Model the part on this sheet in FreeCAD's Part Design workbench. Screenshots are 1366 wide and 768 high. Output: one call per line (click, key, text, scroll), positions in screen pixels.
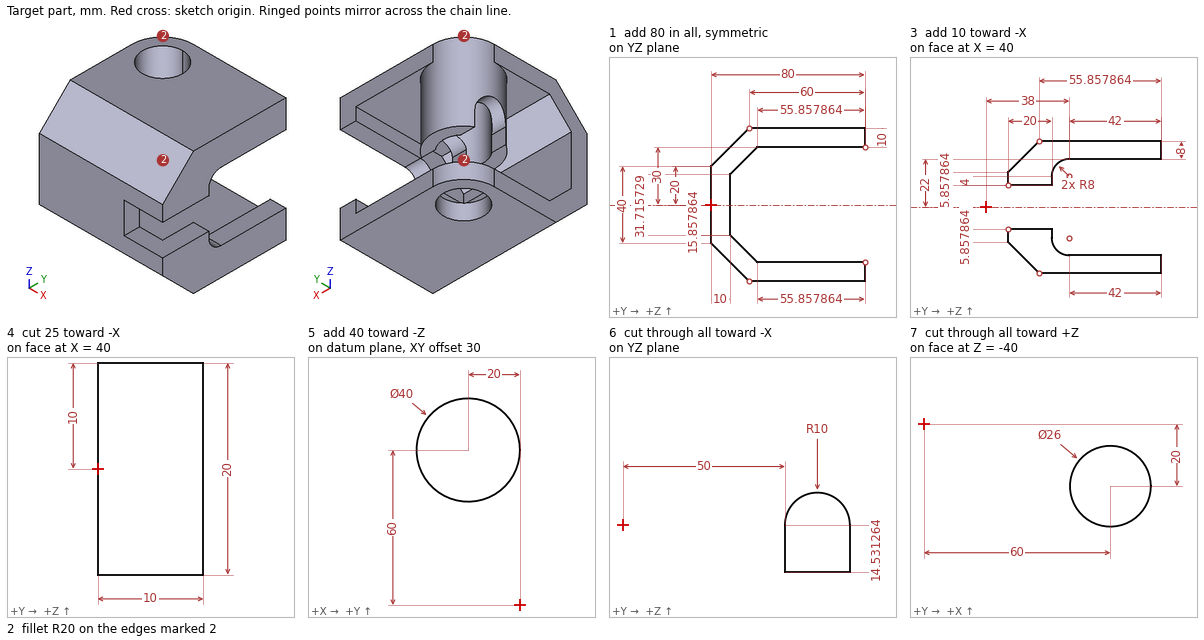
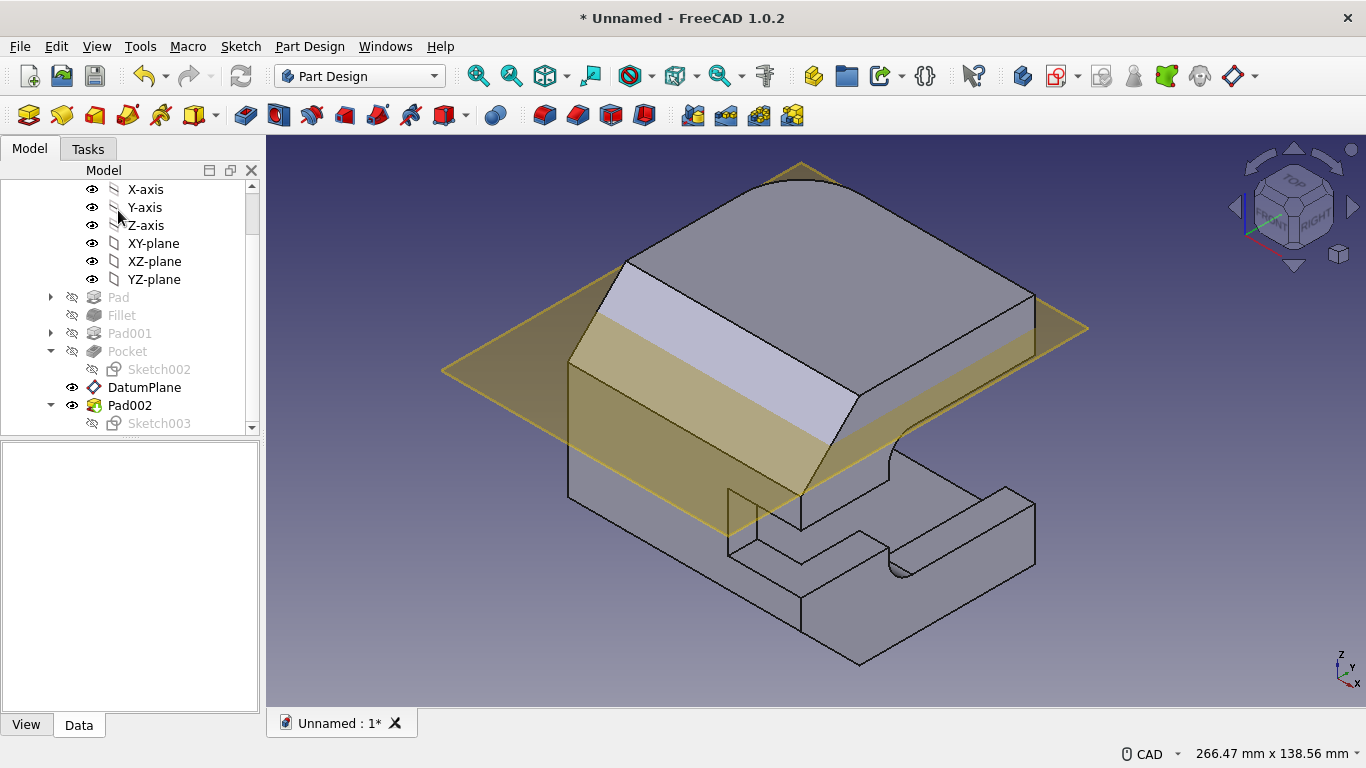
click(117, 387)
key(space)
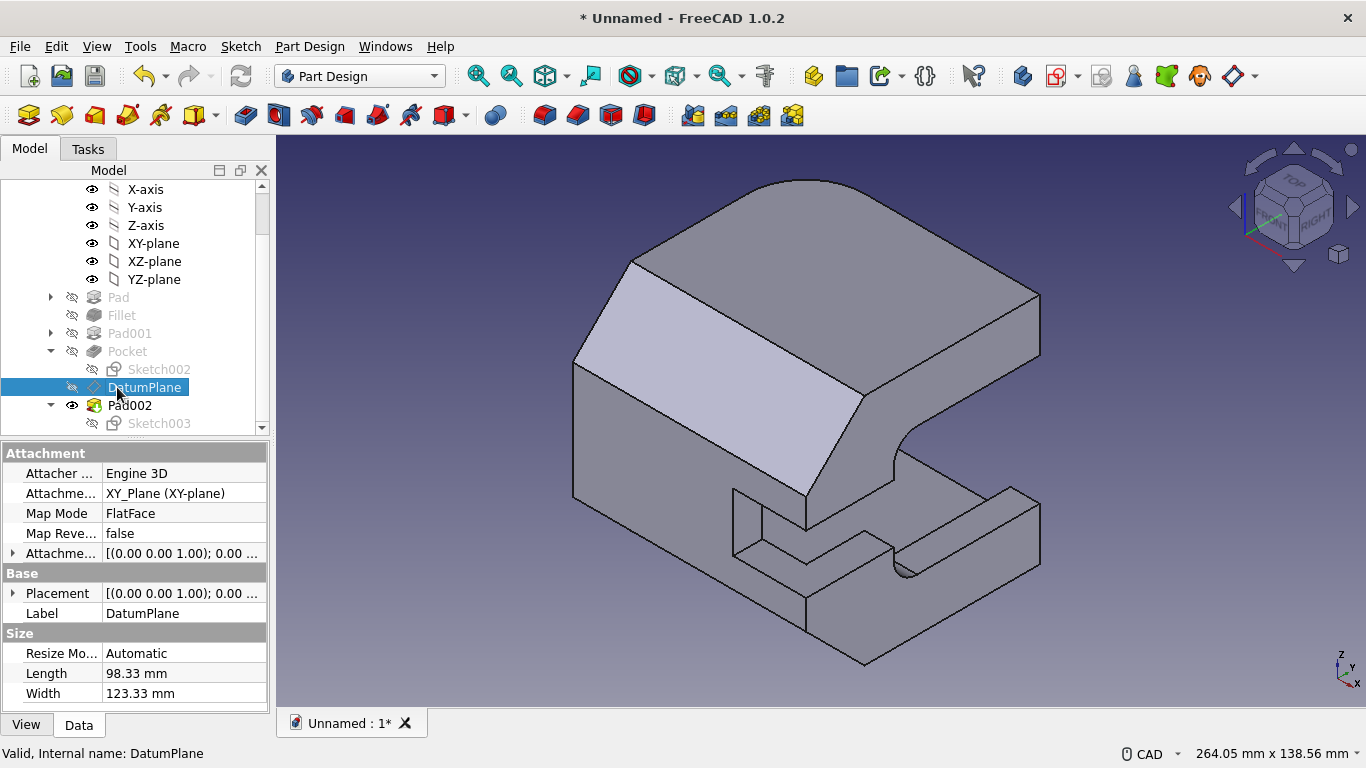
click(316, 667)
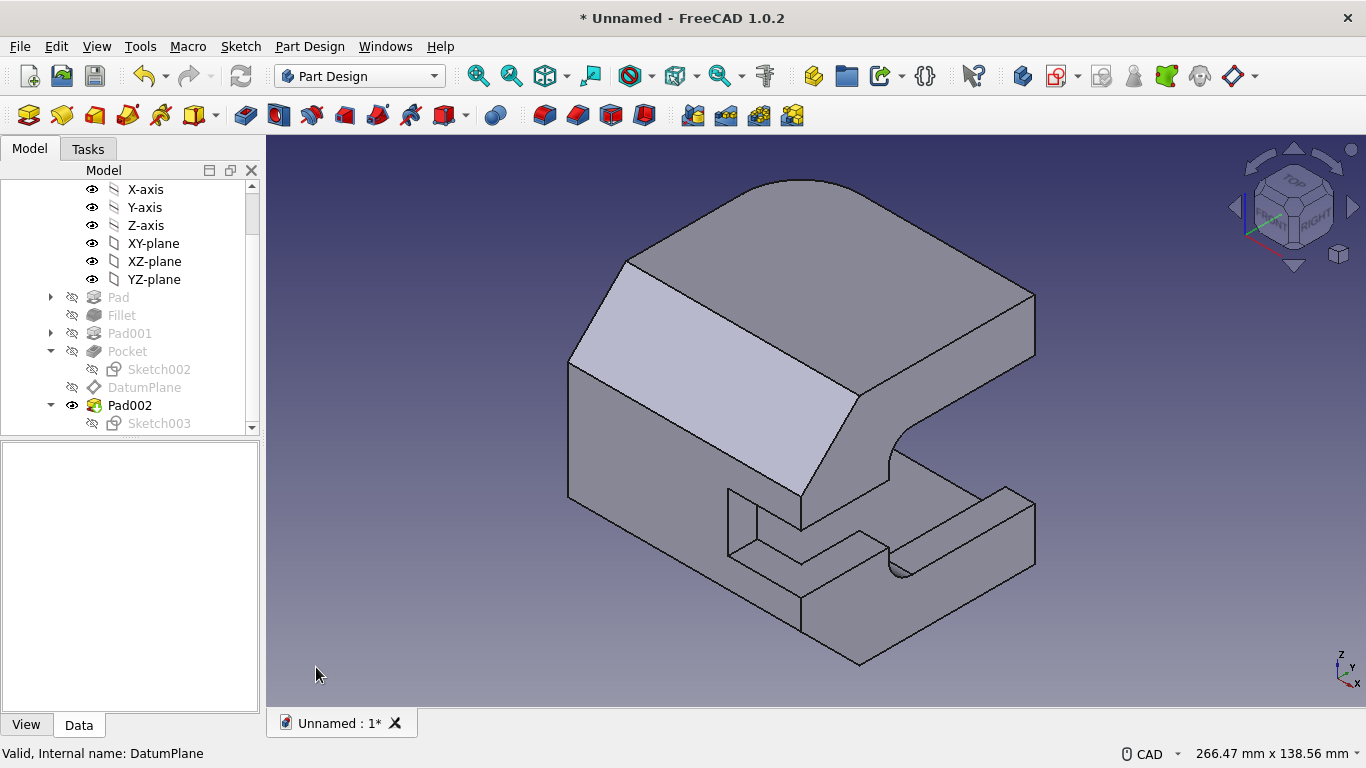
click(1056, 76)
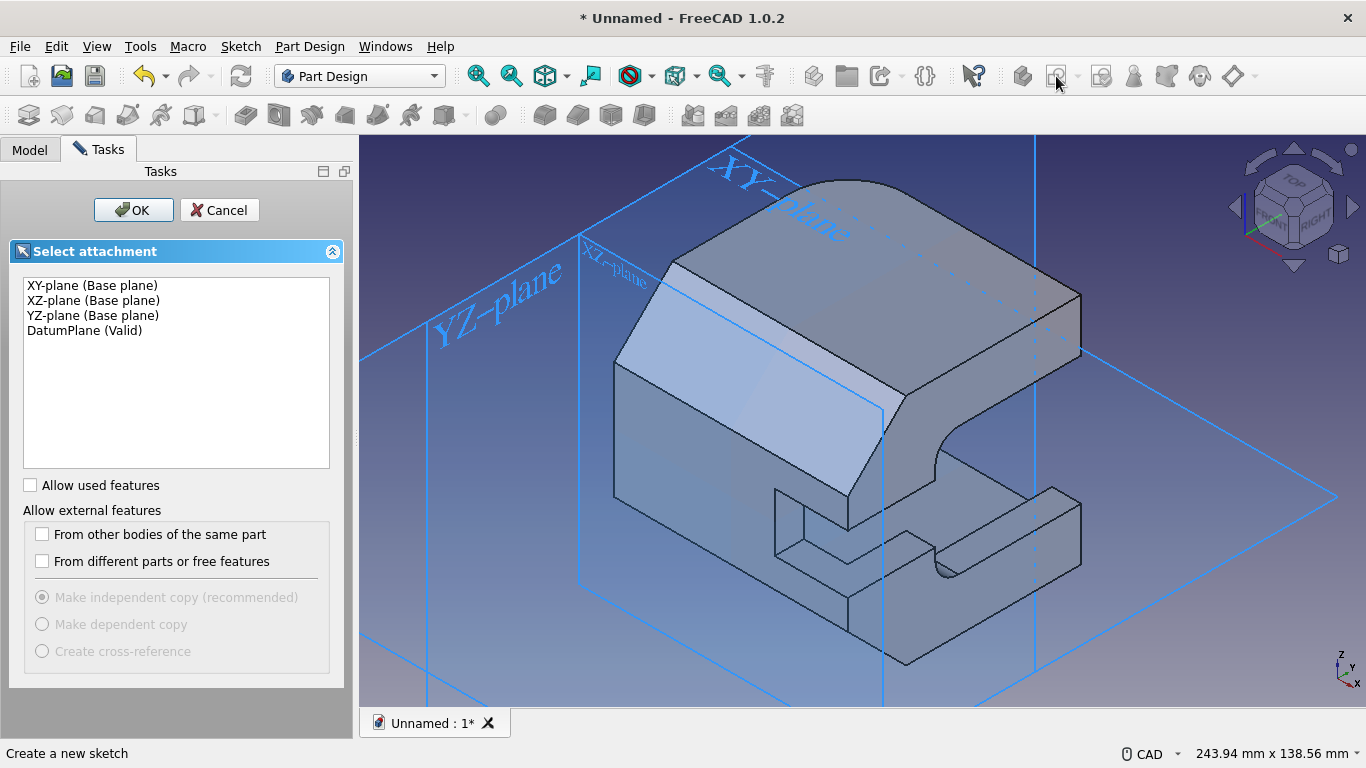
click(84, 316)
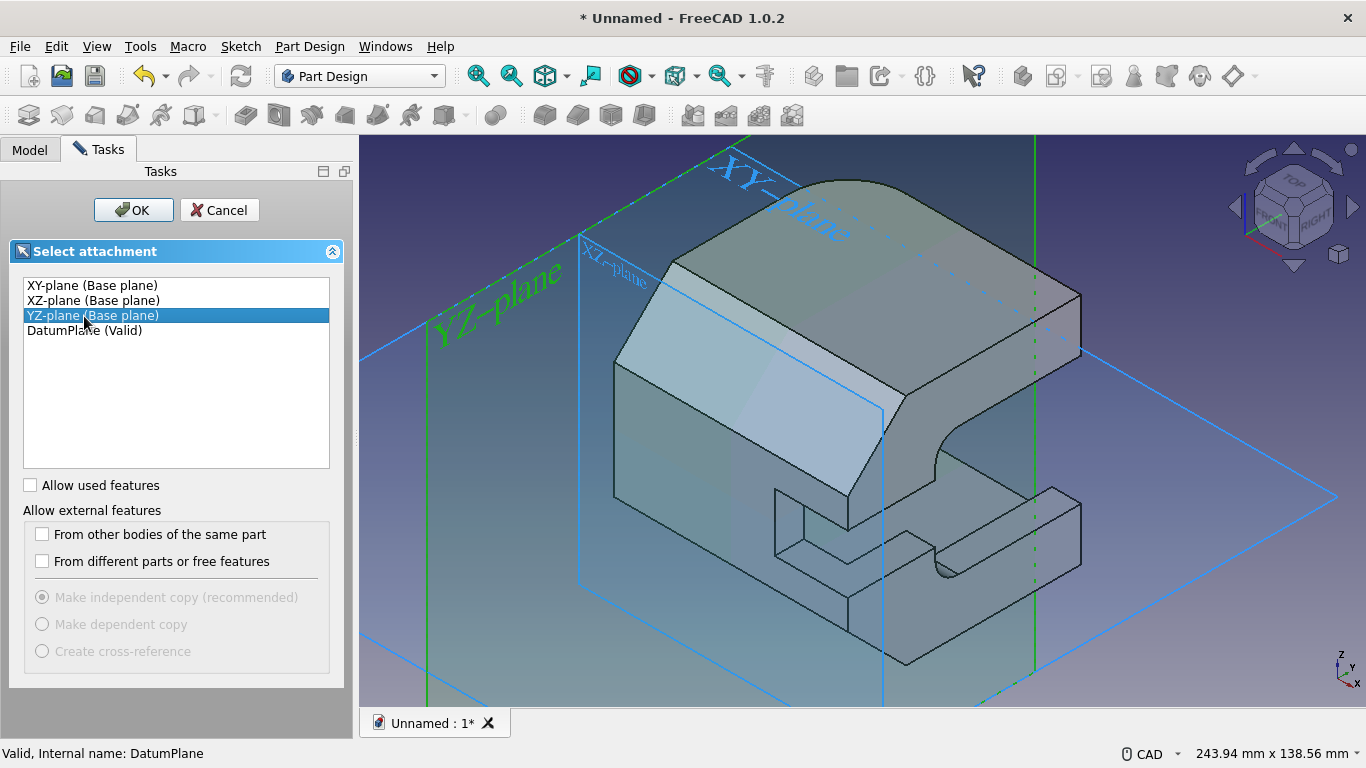
click(134, 210)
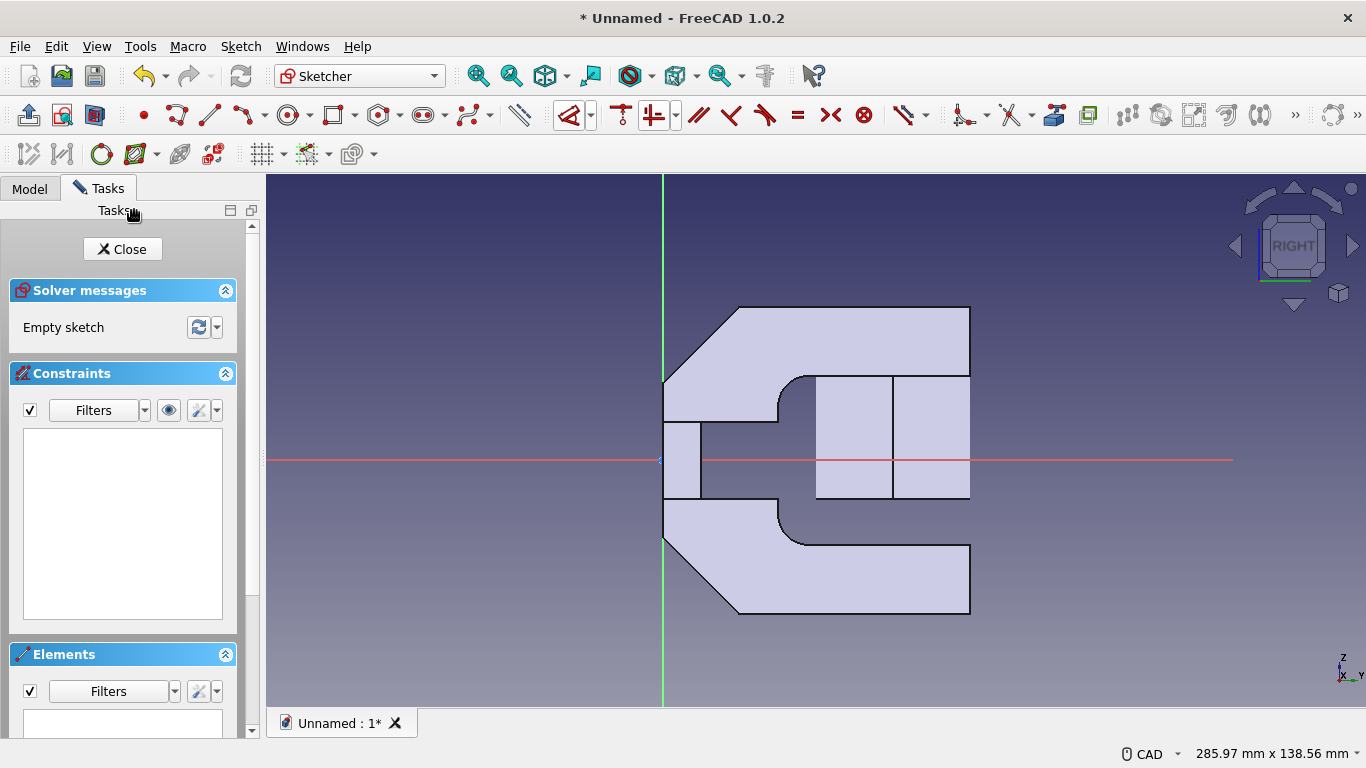
click(95, 116)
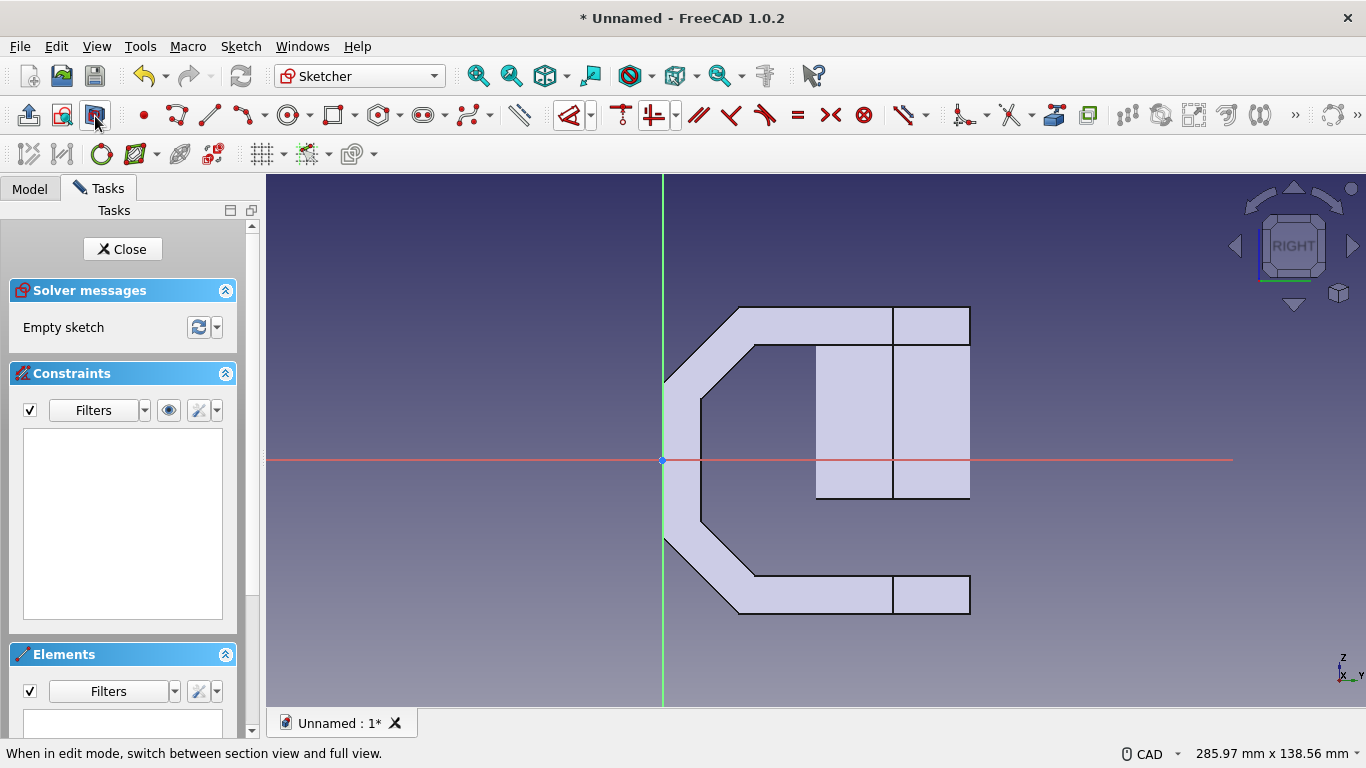
scroll(956, 481, up, 6)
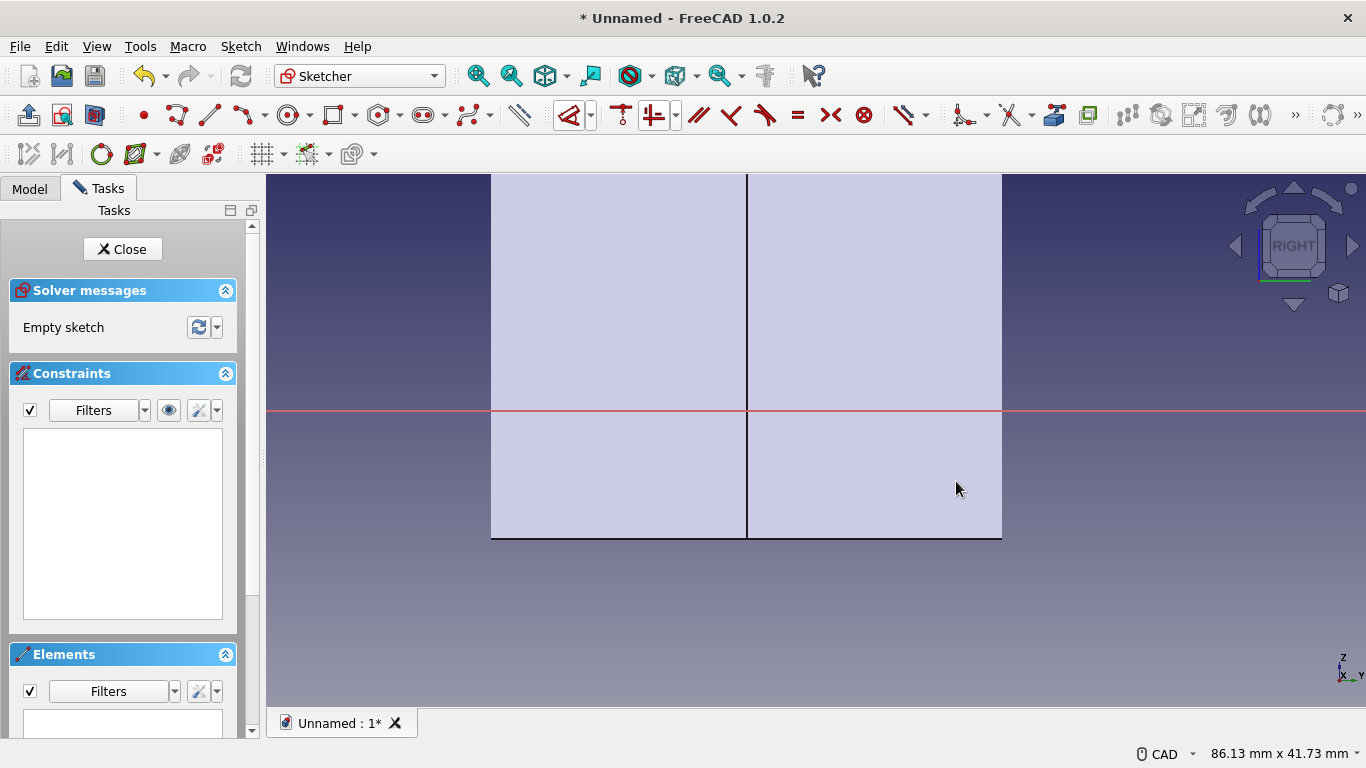
click(177, 116)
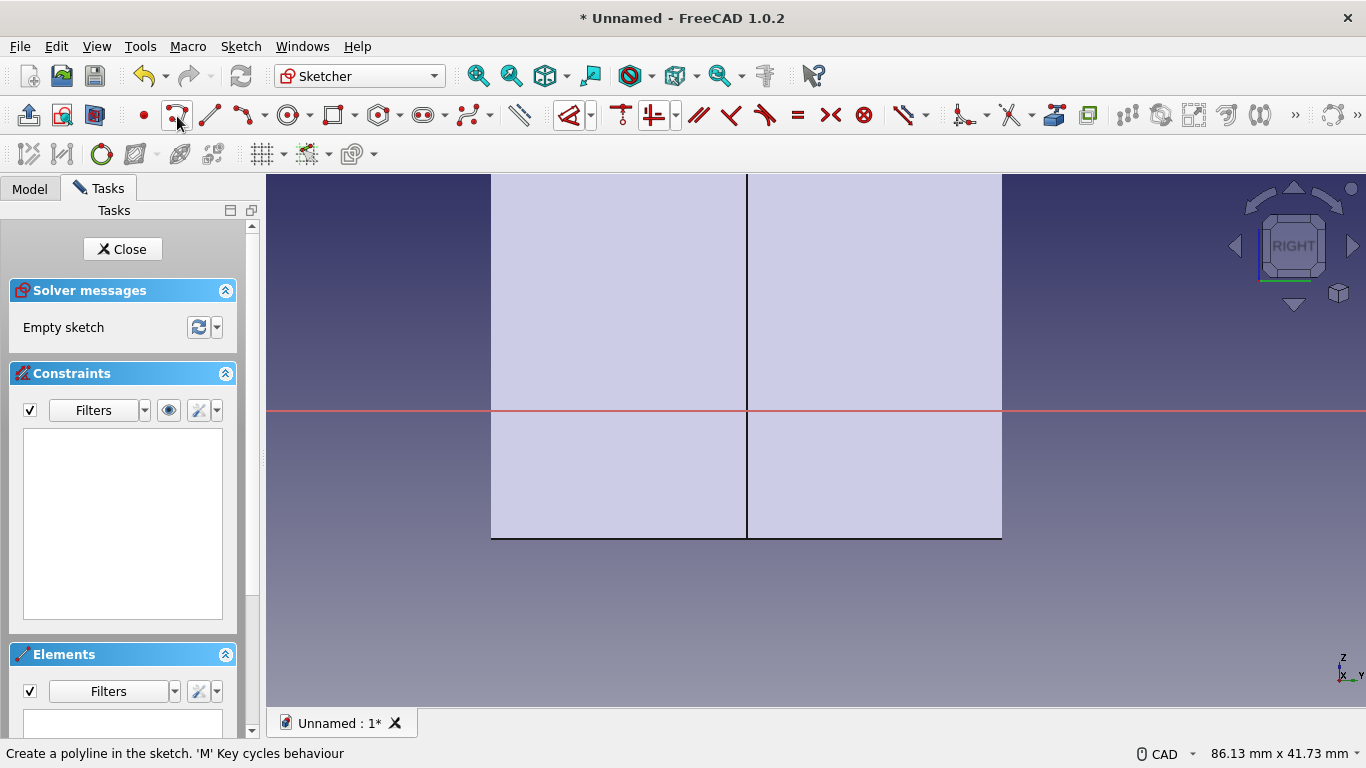
click(619, 411)
click(619, 597)
click(874, 597)
click(874, 411)
right_click(874, 411)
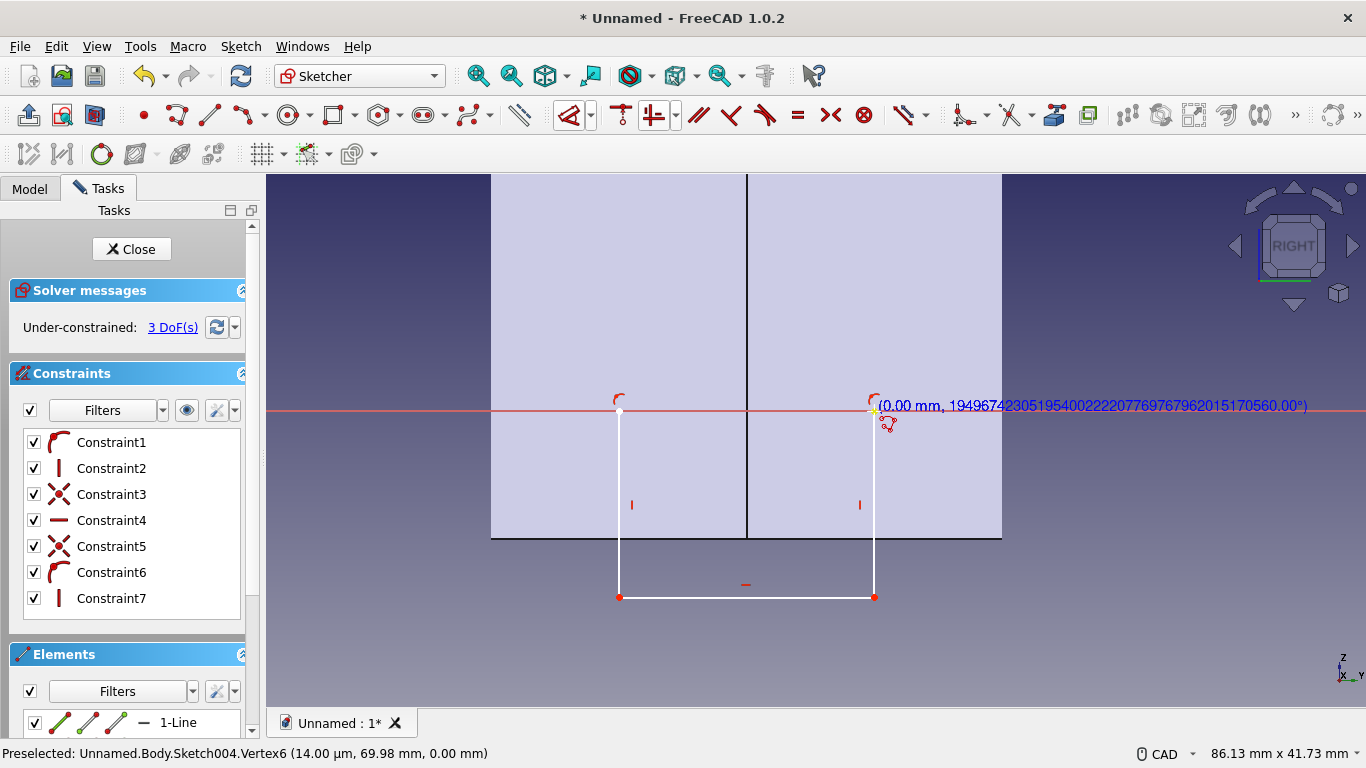
click(242, 116)